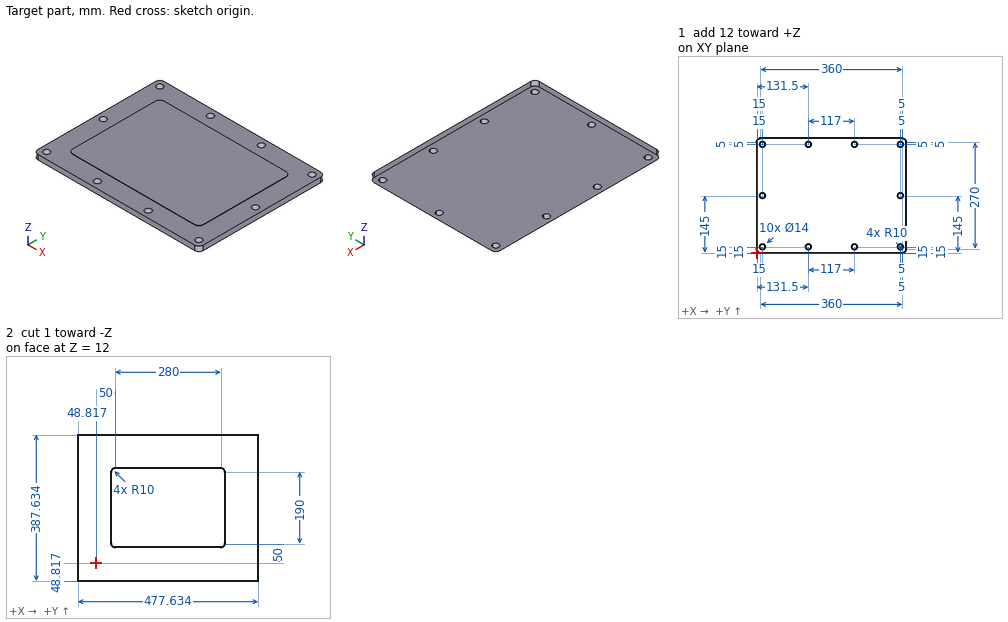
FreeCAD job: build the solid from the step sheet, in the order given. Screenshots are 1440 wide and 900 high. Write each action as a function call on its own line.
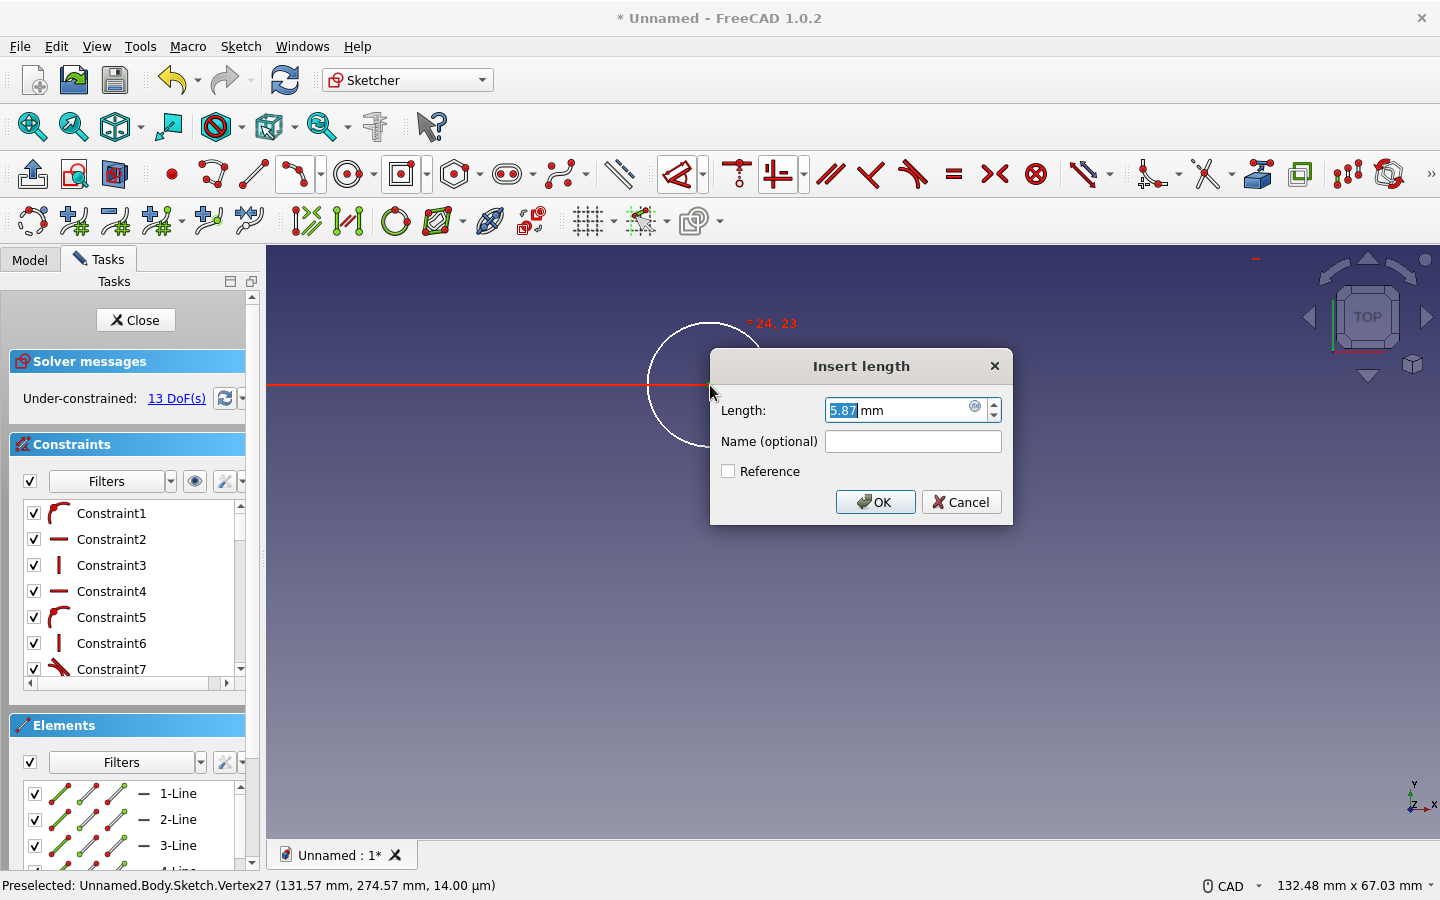
text(5)
key(Return)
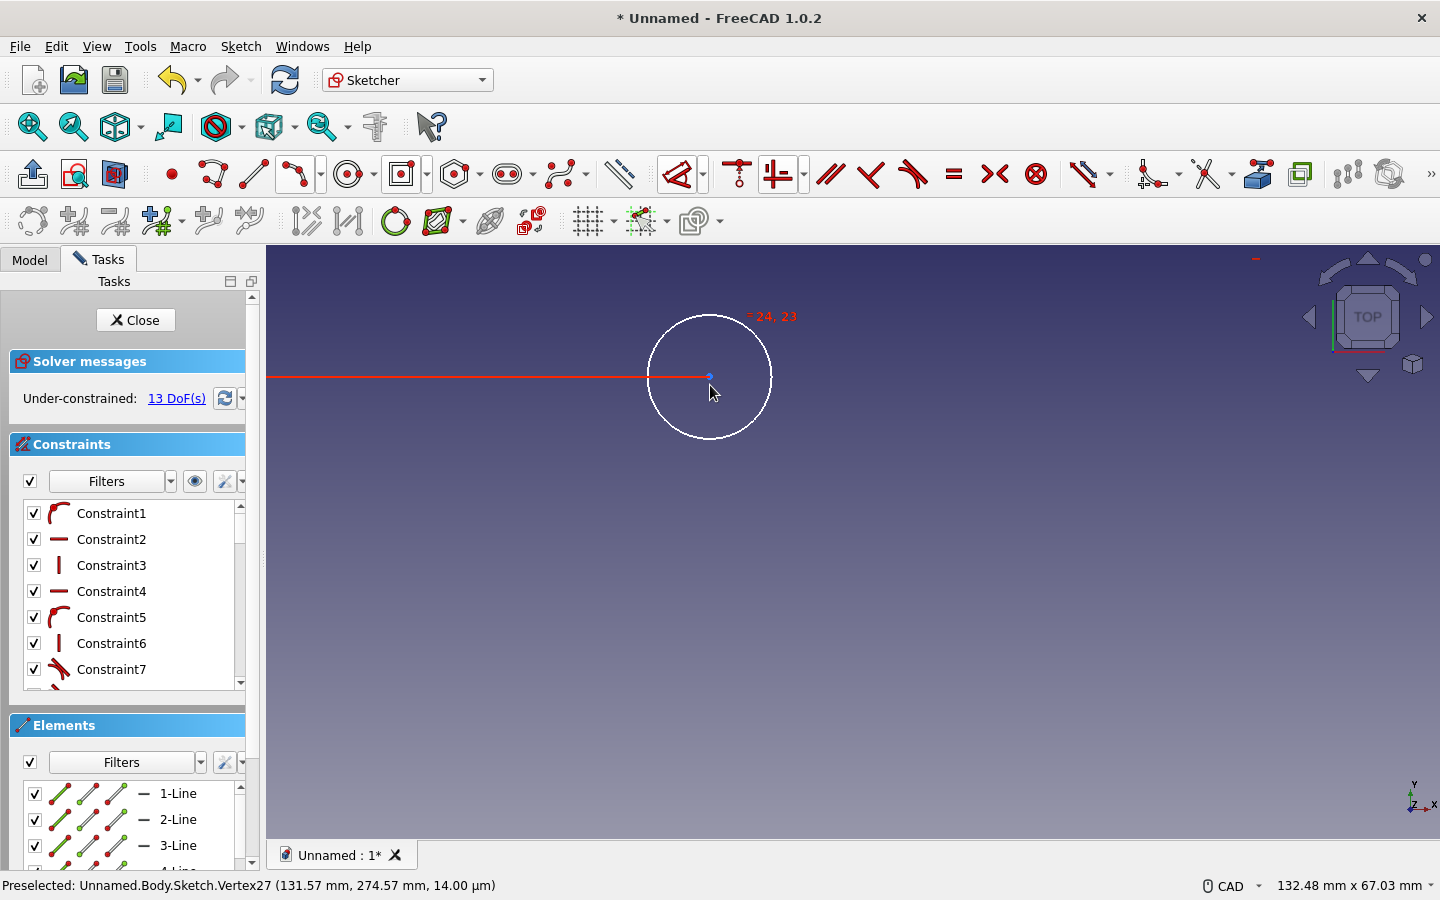
scroll(715, 387, down, 10)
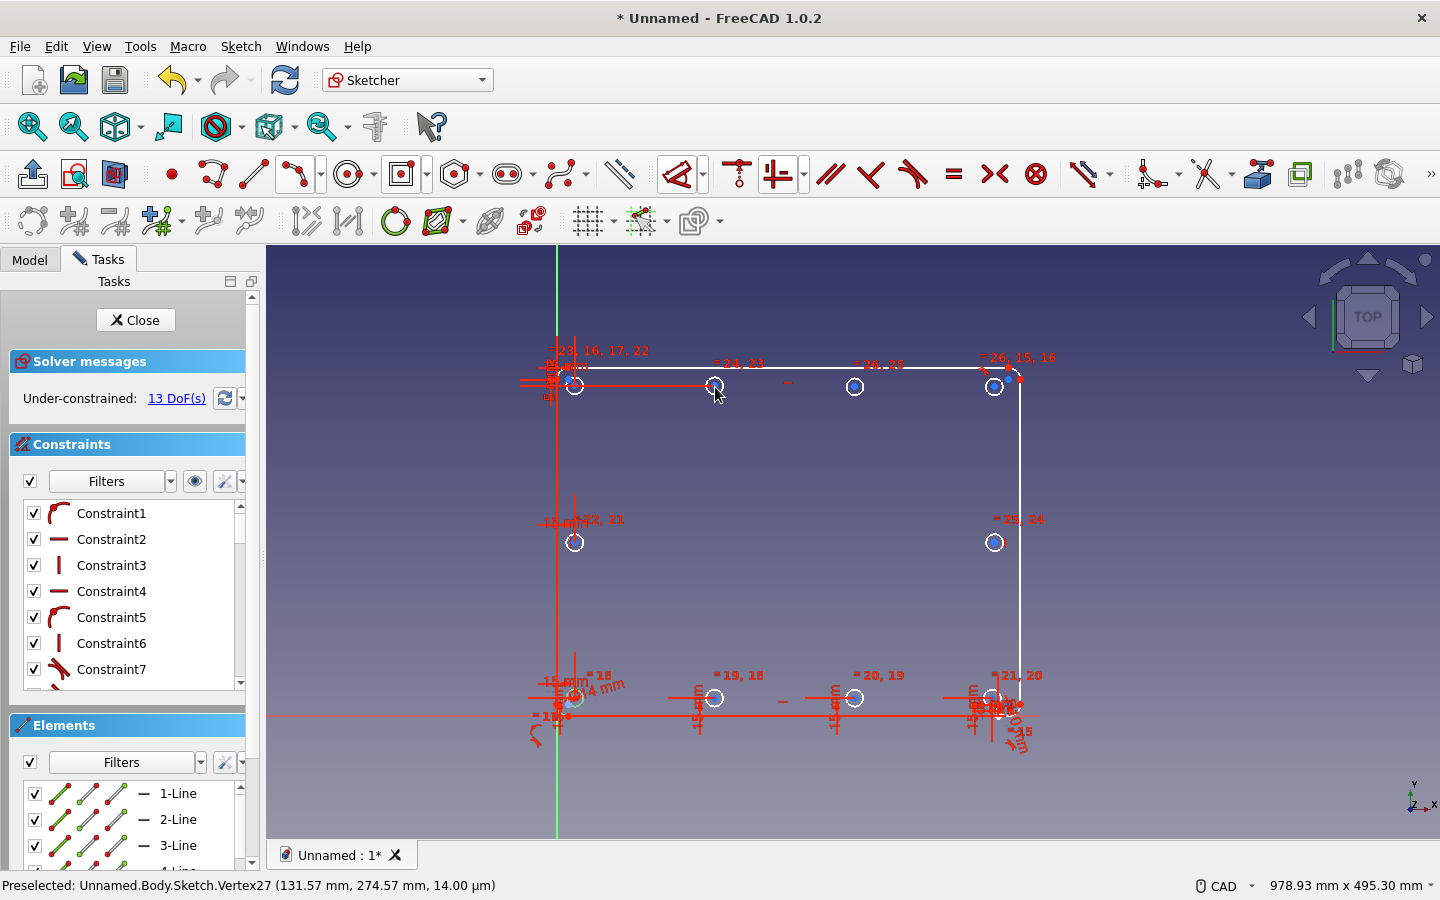
scroll(998, 716, up, 10)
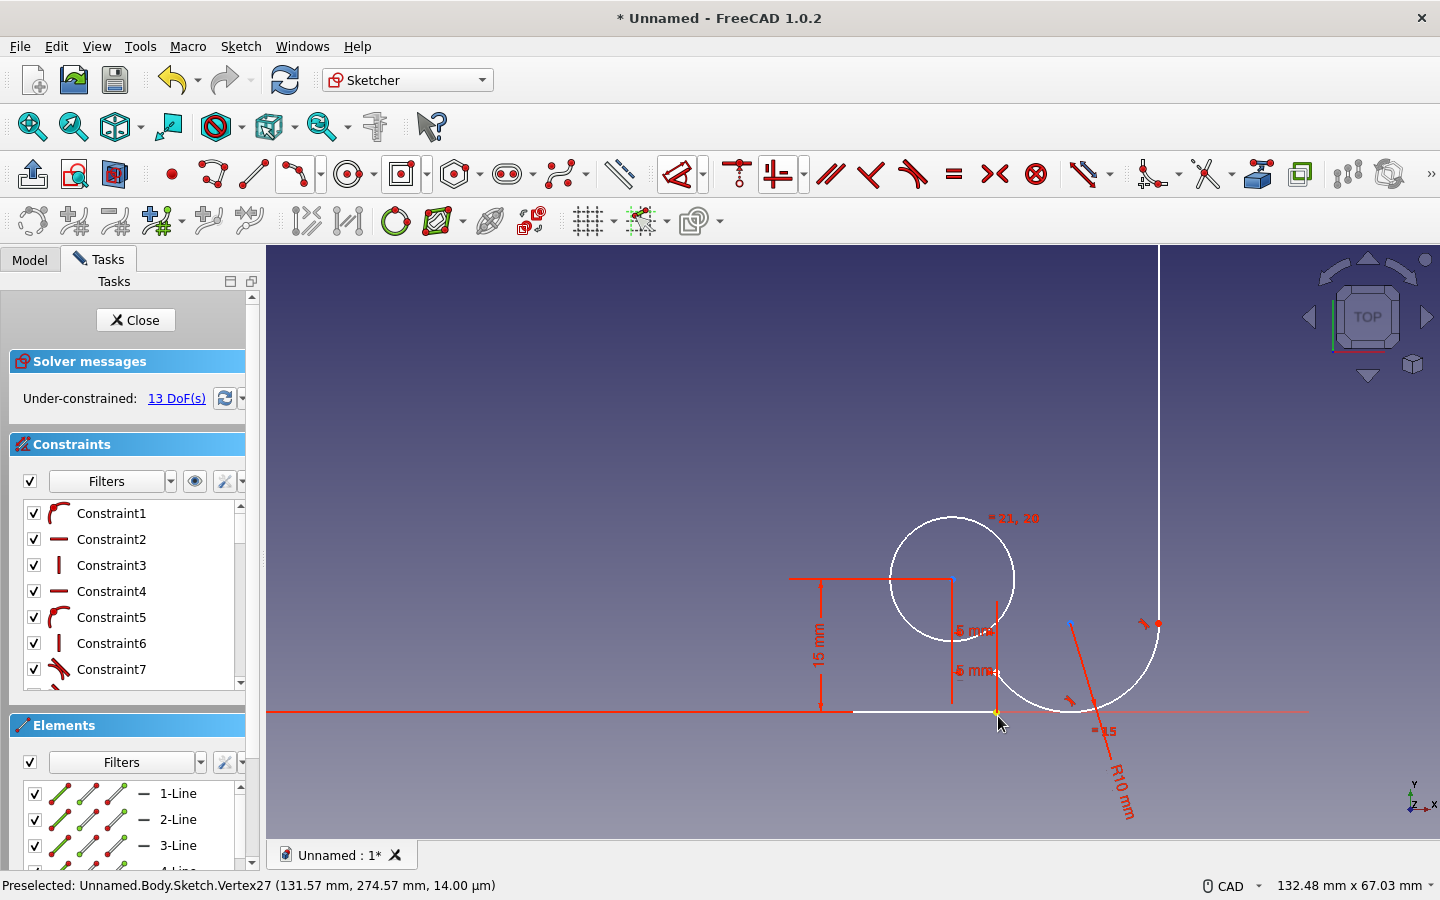
click(997, 712)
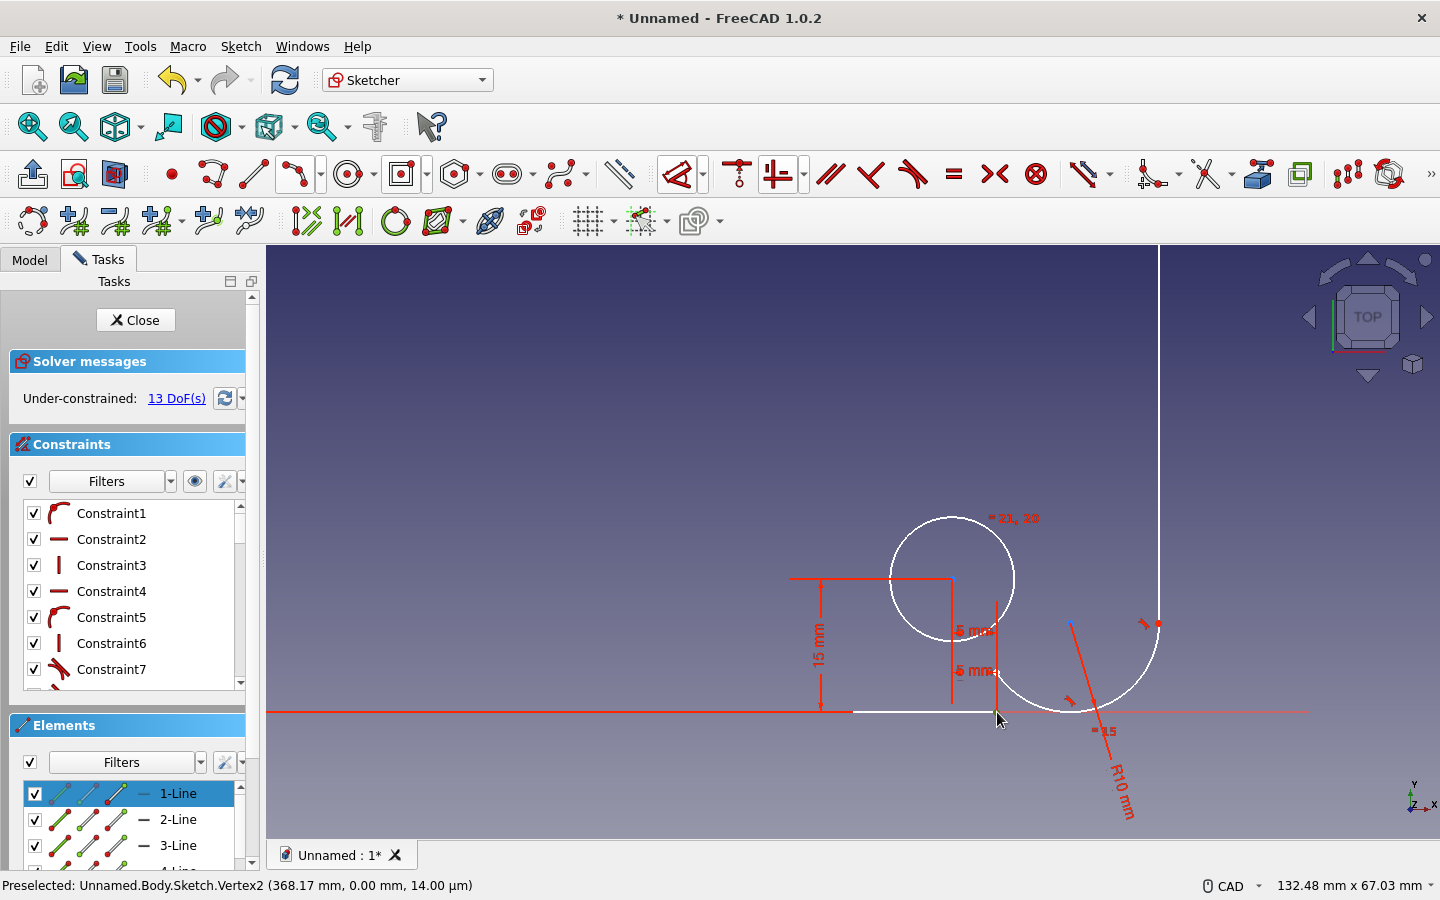
scroll(998, 716, down, 10)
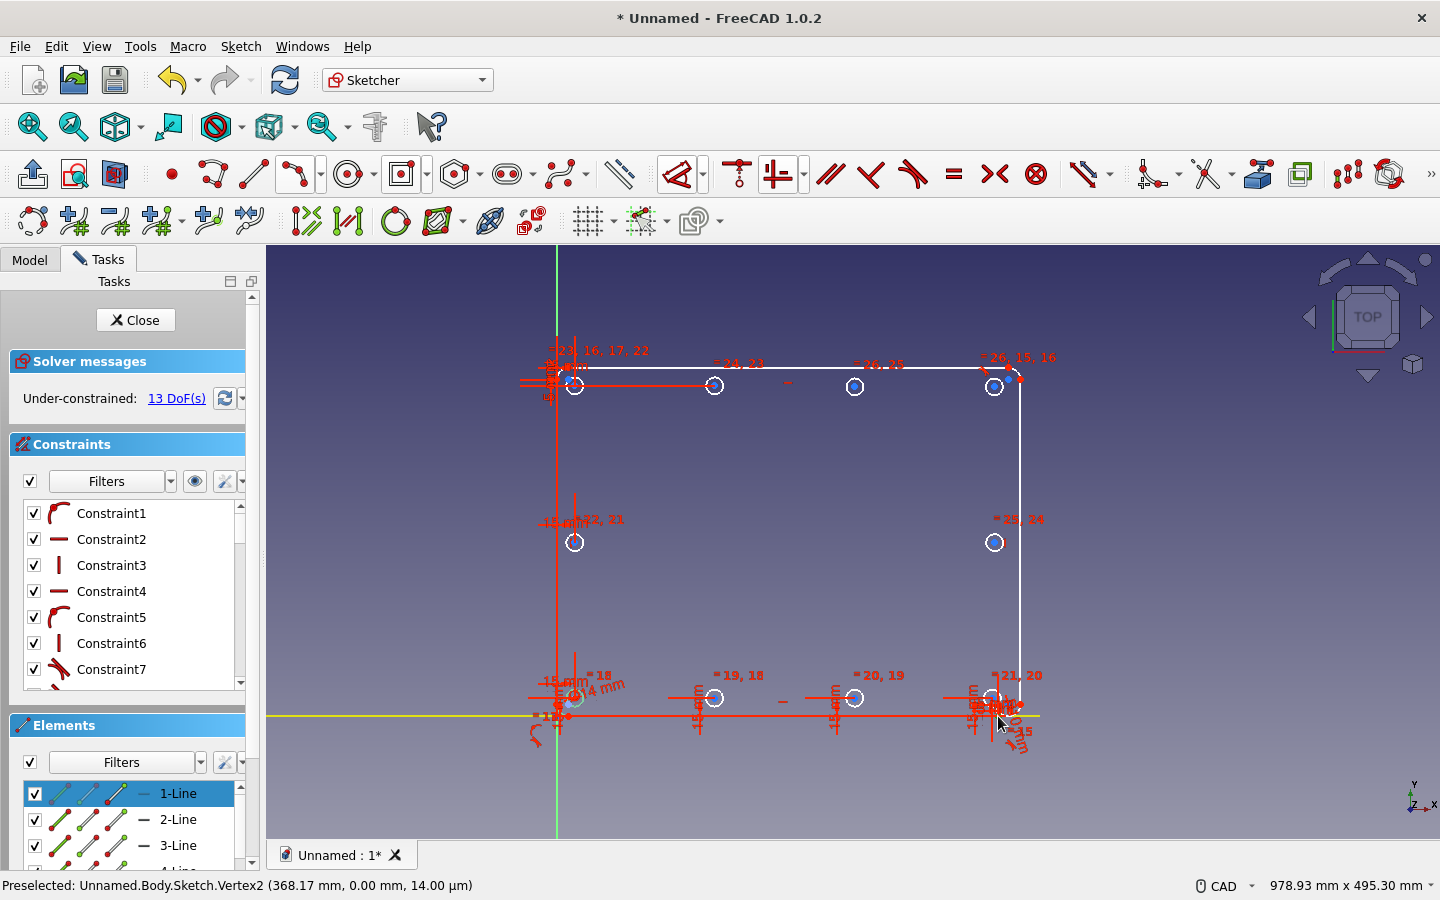
scroll(995, 543, up, 10)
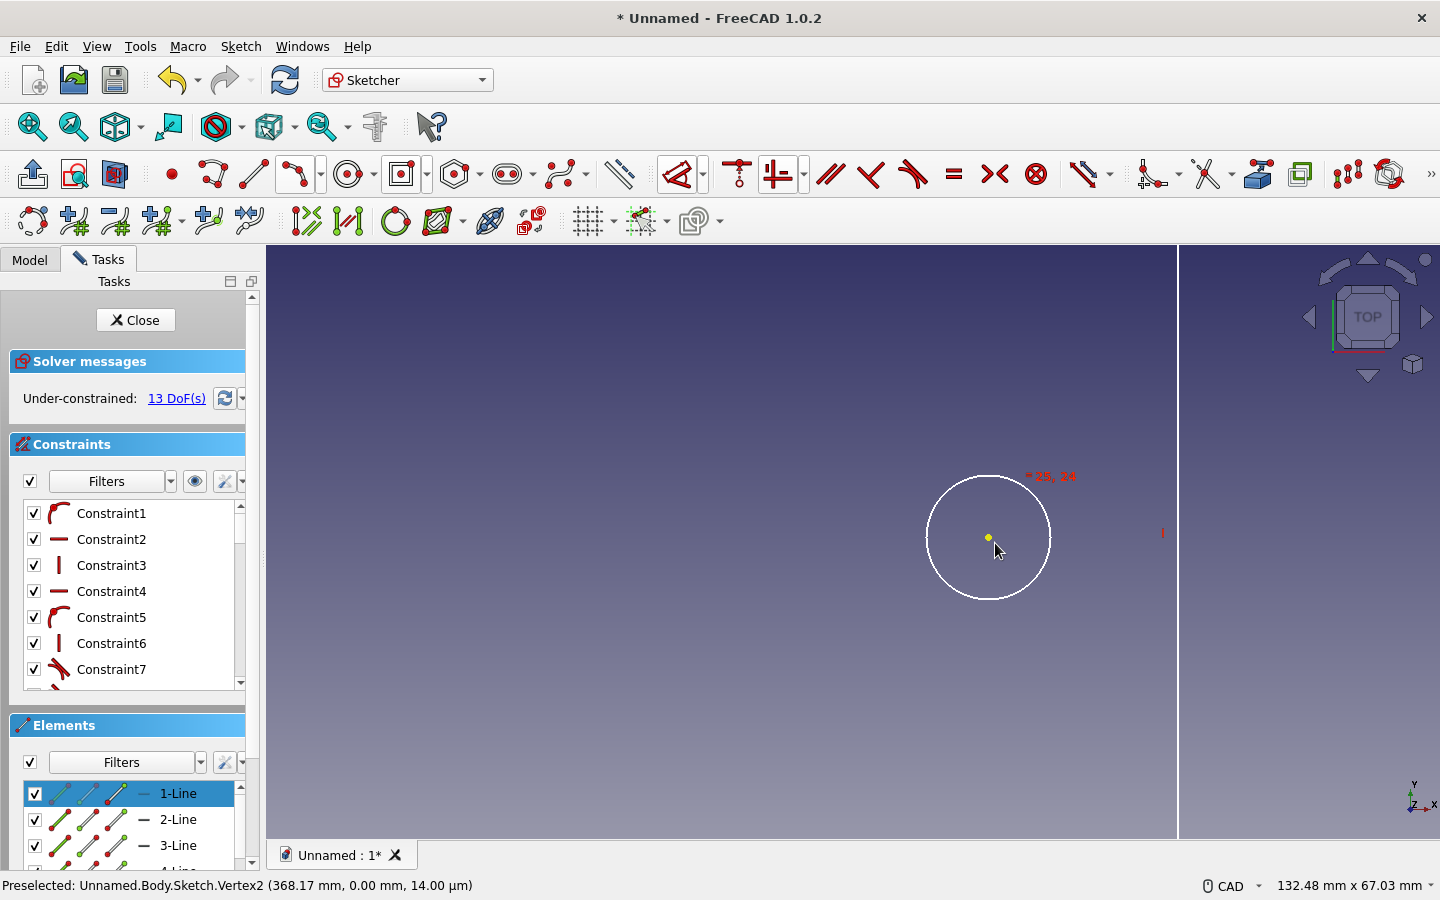
click(988, 537)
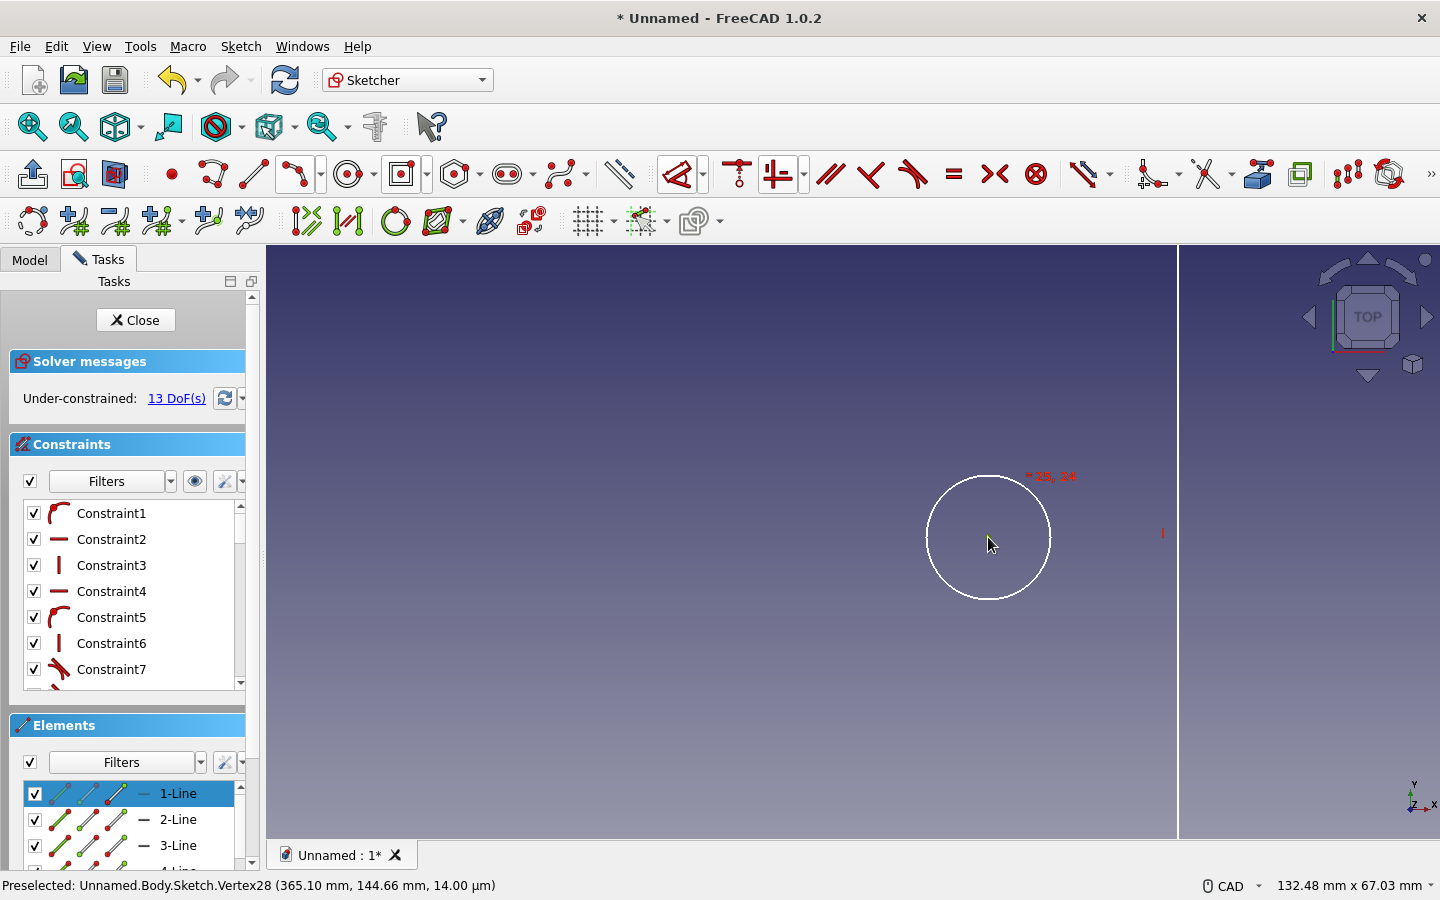
click(702, 174)